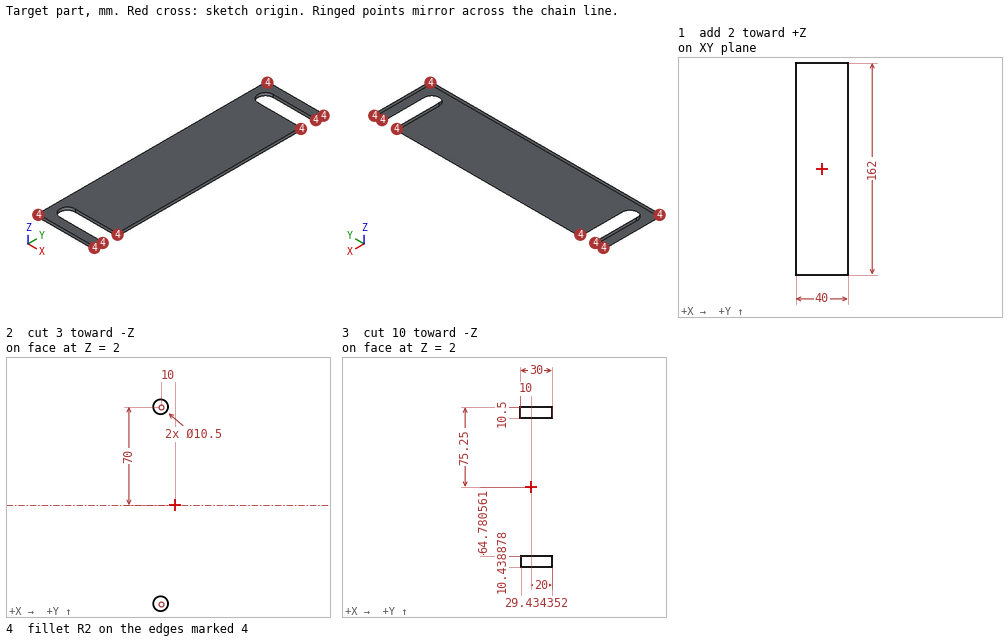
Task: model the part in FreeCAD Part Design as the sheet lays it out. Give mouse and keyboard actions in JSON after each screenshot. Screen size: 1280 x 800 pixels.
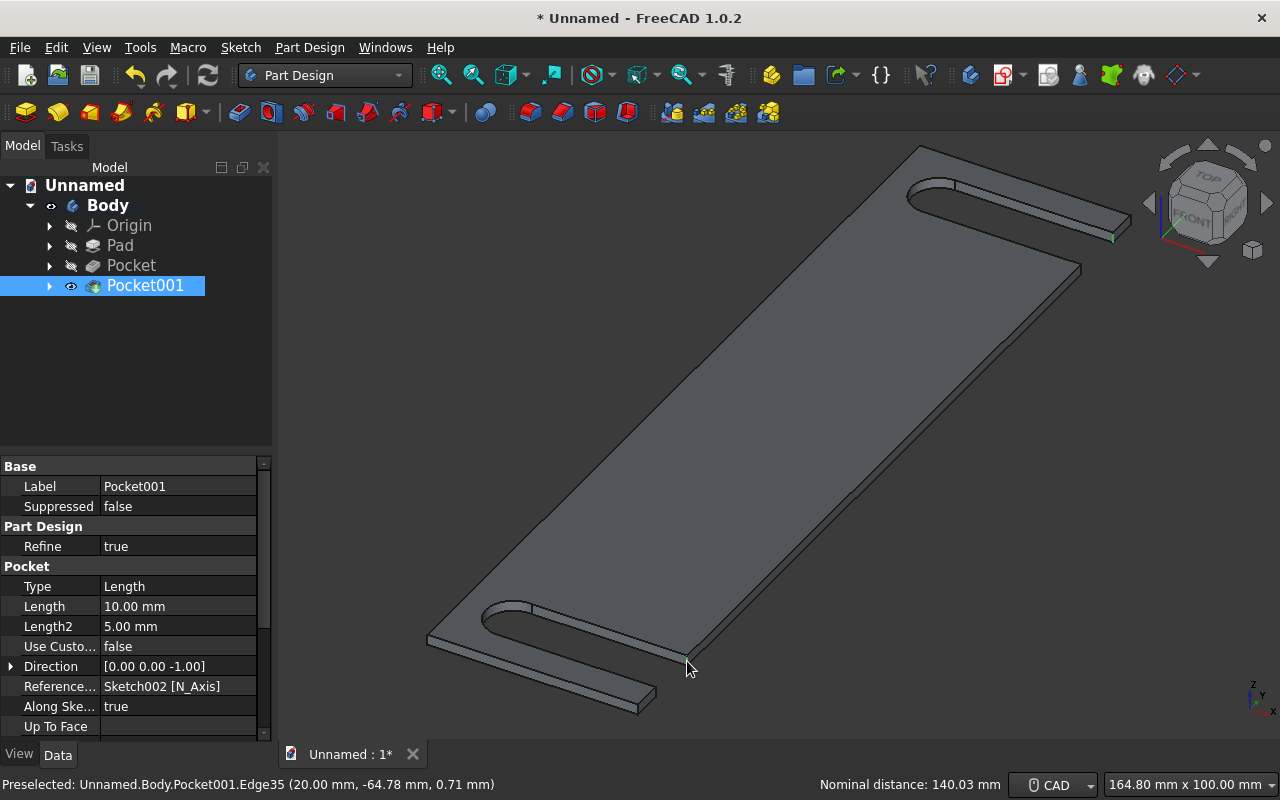
{"action": "left_click", "coordinate": [638, 710], "text": "ctrl"}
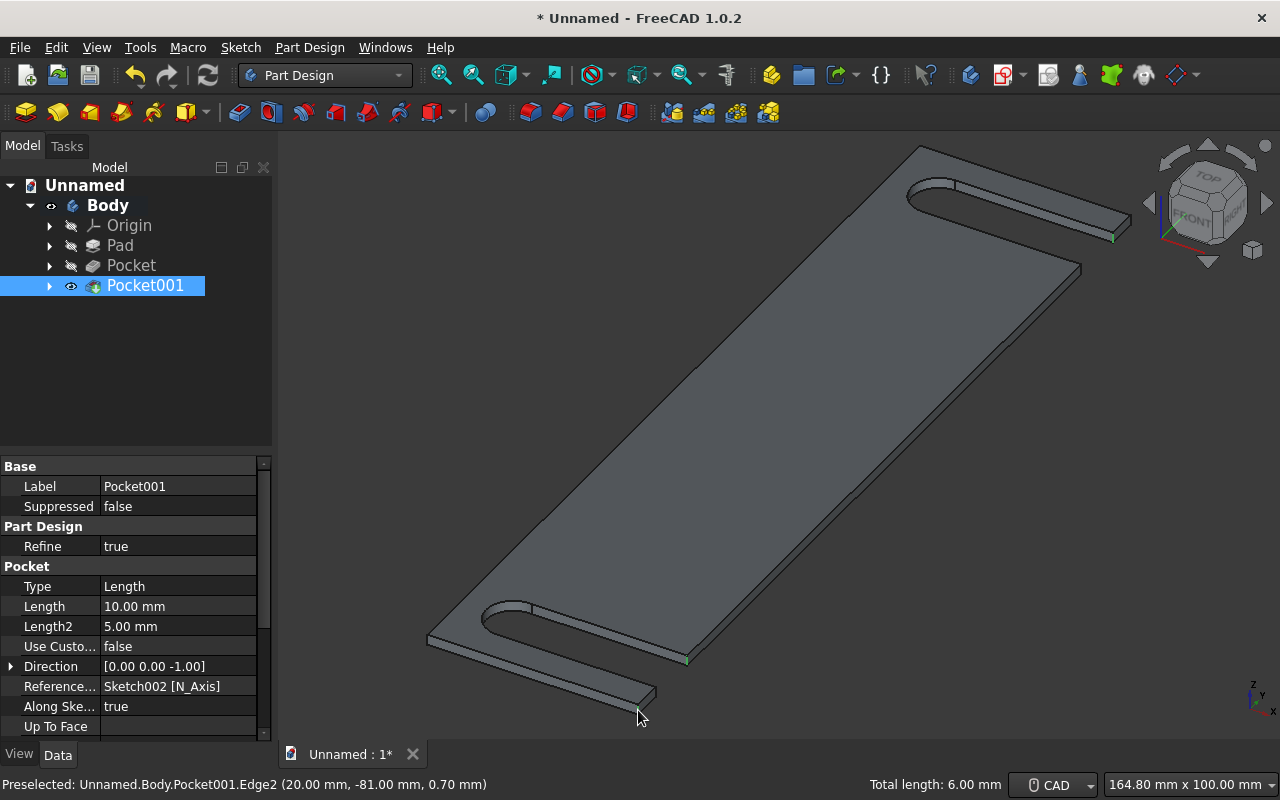
{"action": "scroll", "coordinate": [1081, 268], "scroll_direction": "up", "scroll_amount": 6}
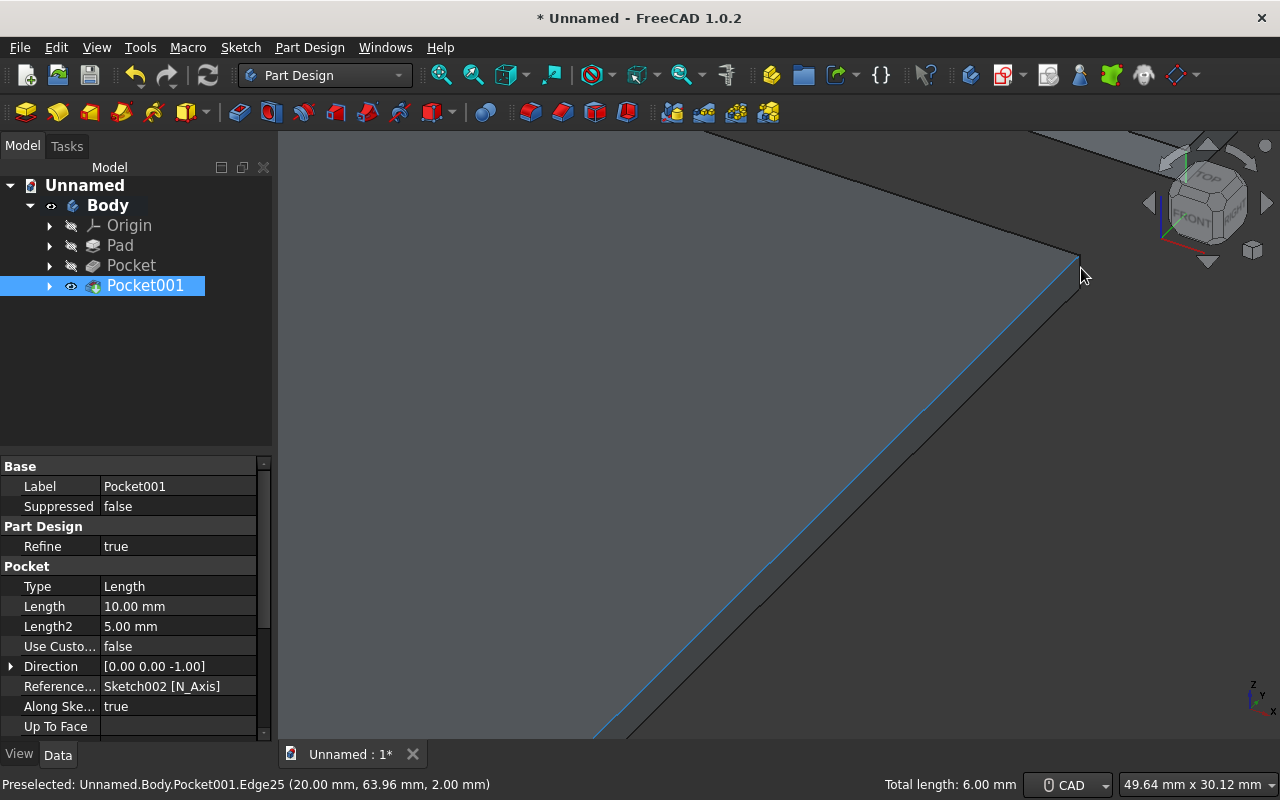
{"action": "left_click", "coordinate": [442, 76]}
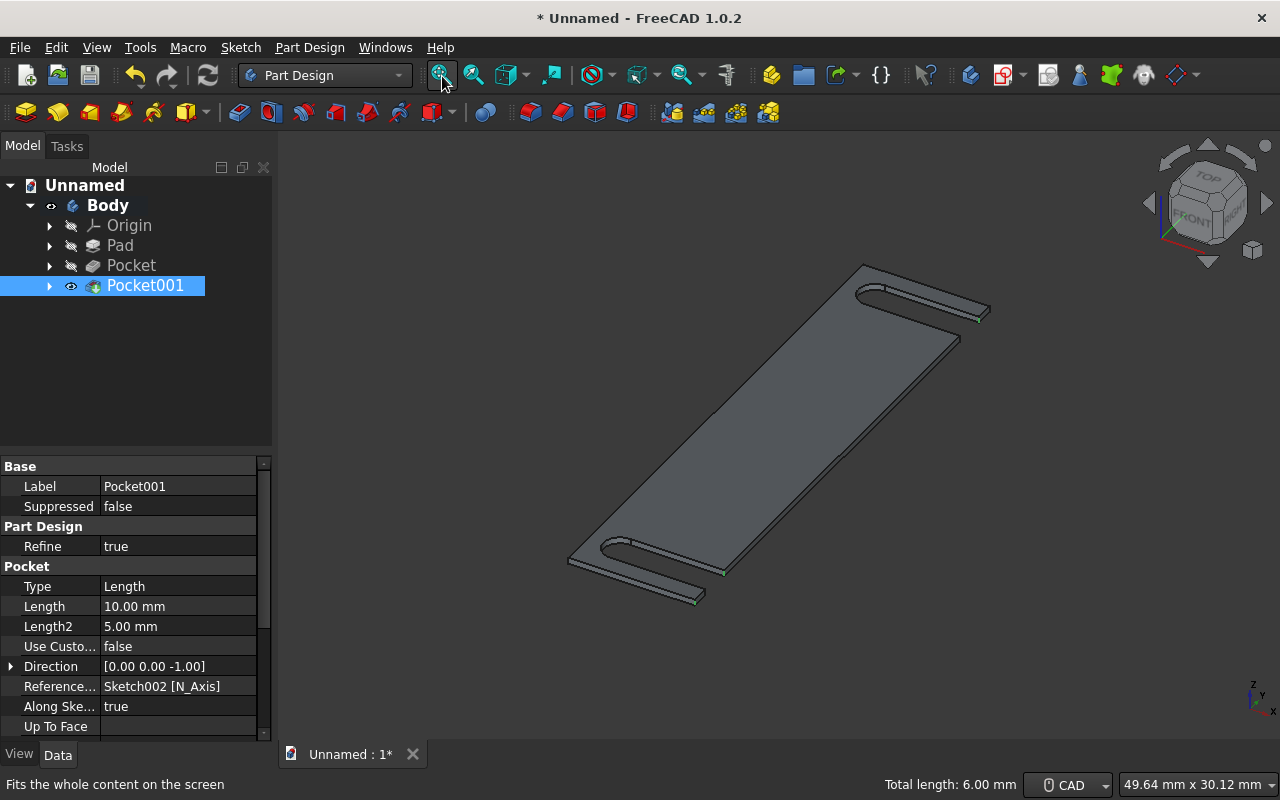
{"action": "key", "text": "0"}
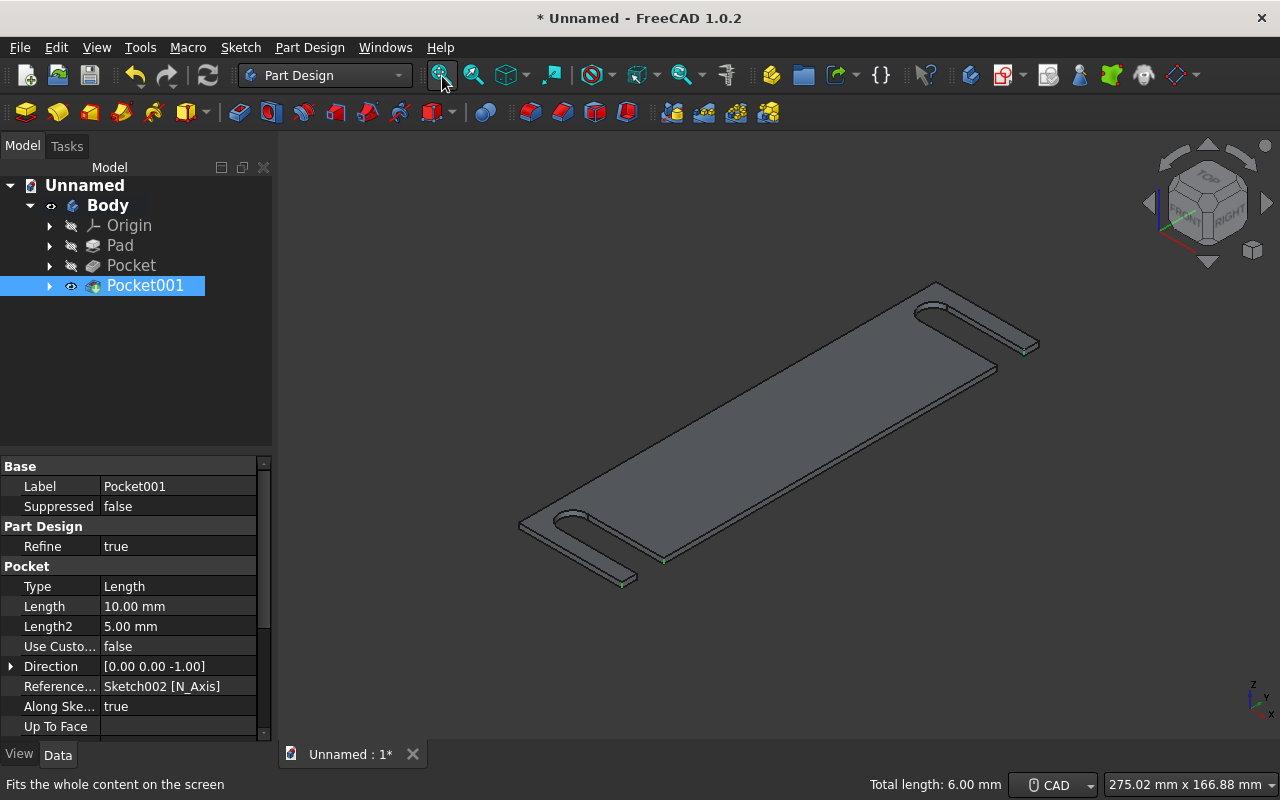
{"action": "scroll", "coordinate": [997, 367], "scroll_direction": "up", "scroll_amount": 9}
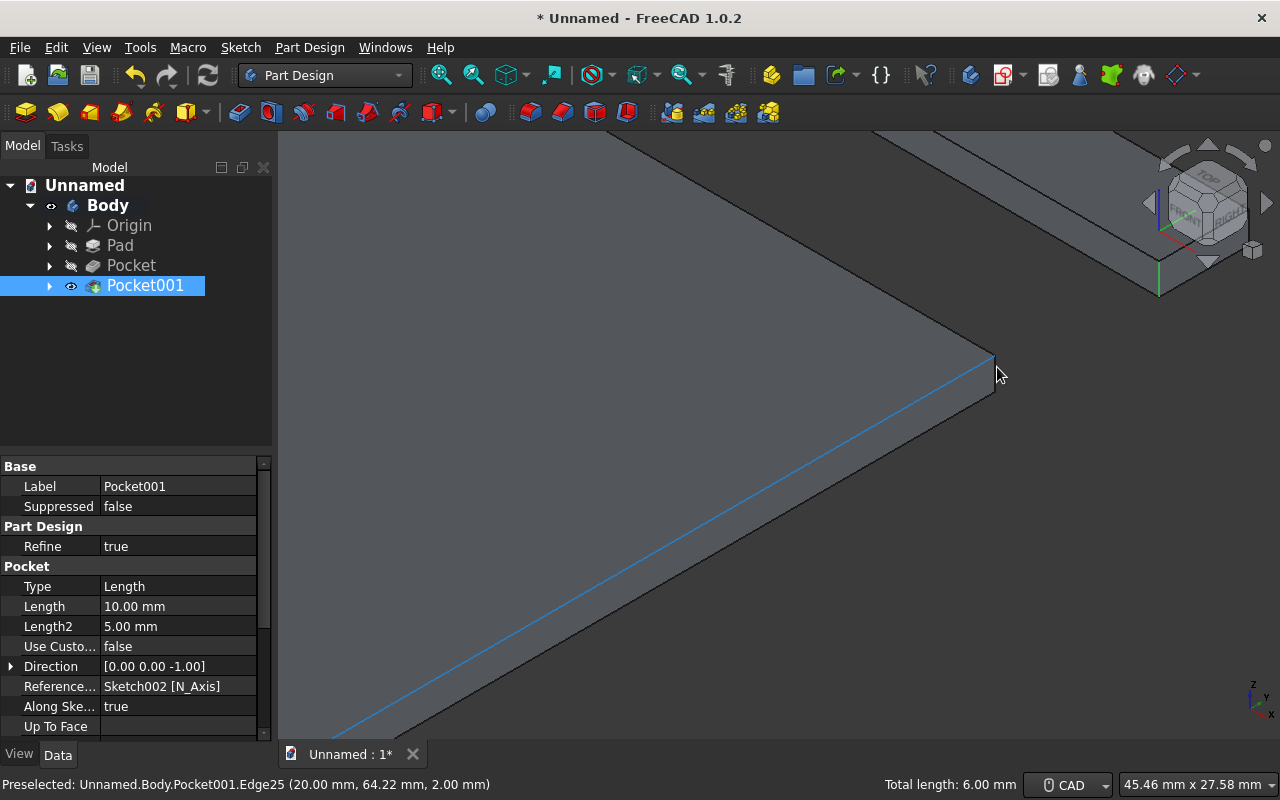
{"action": "left_click", "coordinate": [442, 76]}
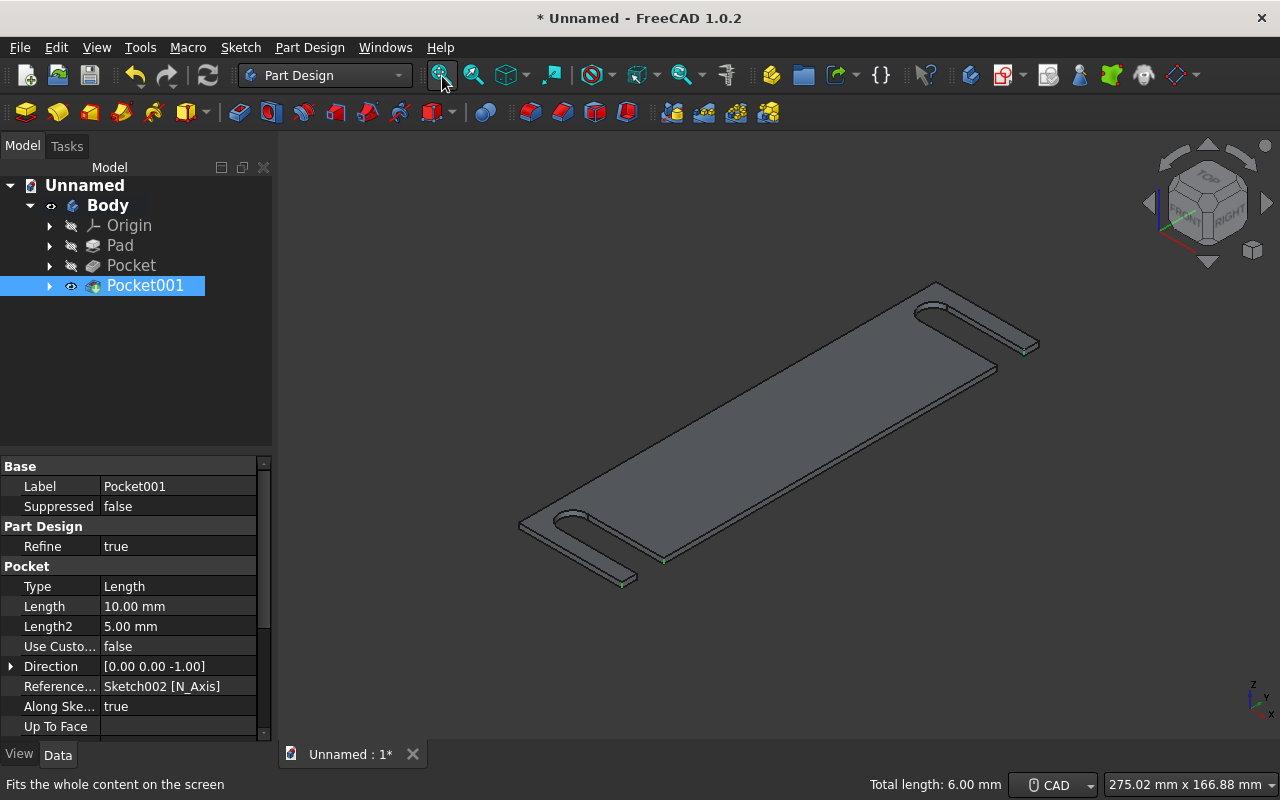
{"action": "key", "text": "2"}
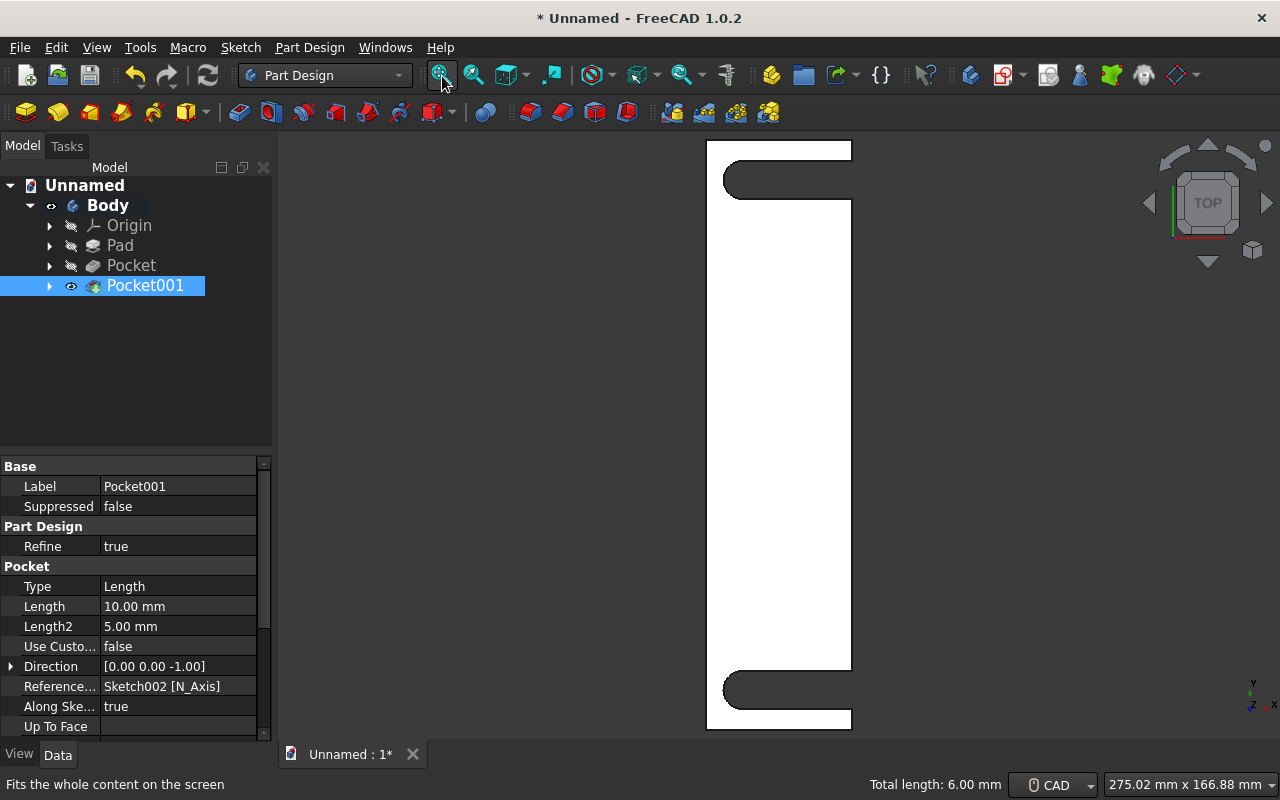
{"action": "scroll", "coordinate": [852, 198], "scroll_direction": "up", "scroll_amount": 9}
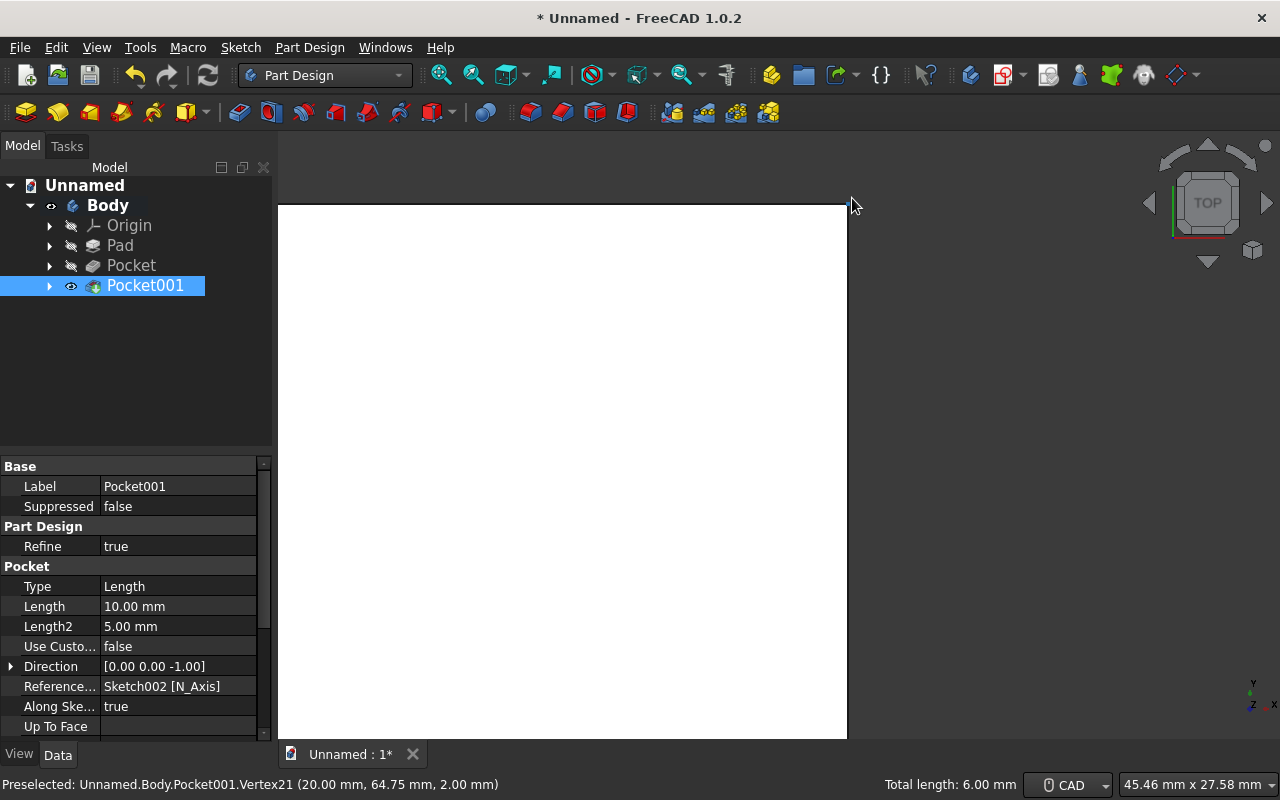
{"action": "left_click", "coordinate": [442, 76]}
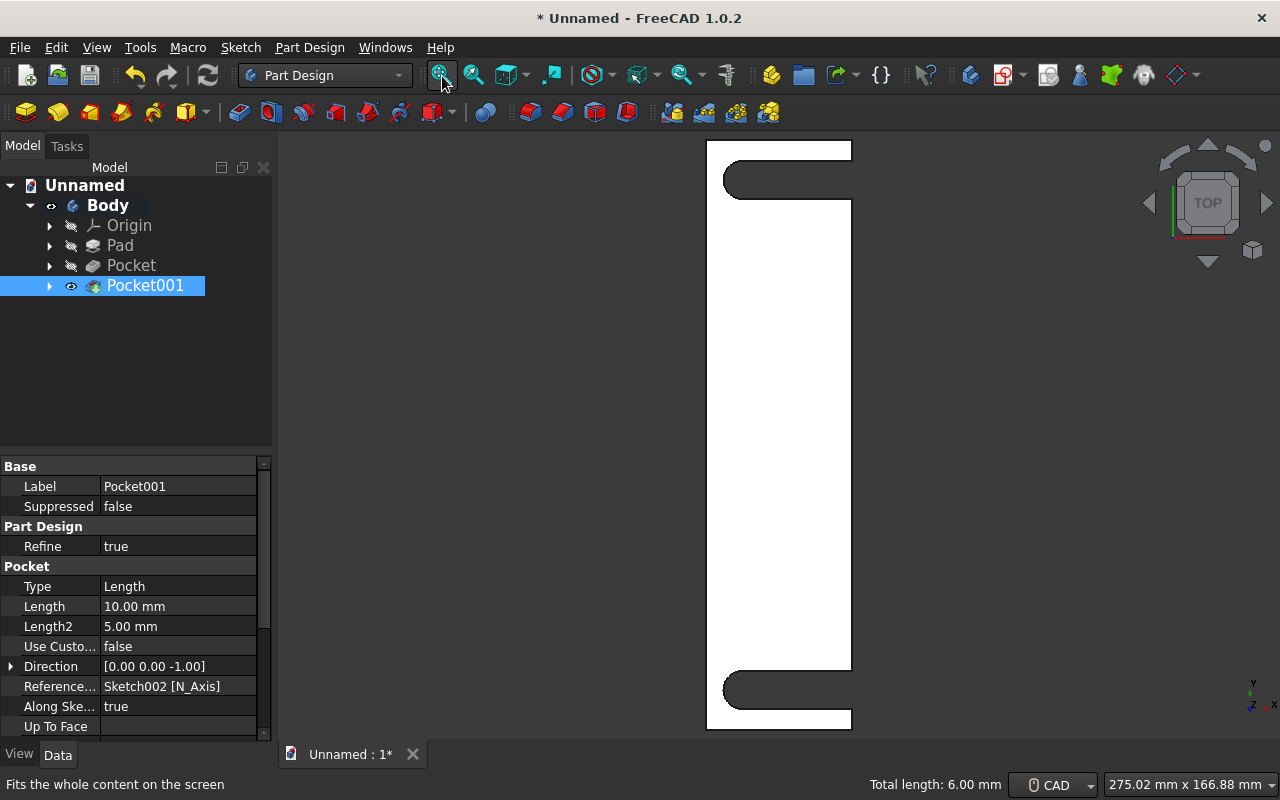
{"action": "key", "text": "1"}